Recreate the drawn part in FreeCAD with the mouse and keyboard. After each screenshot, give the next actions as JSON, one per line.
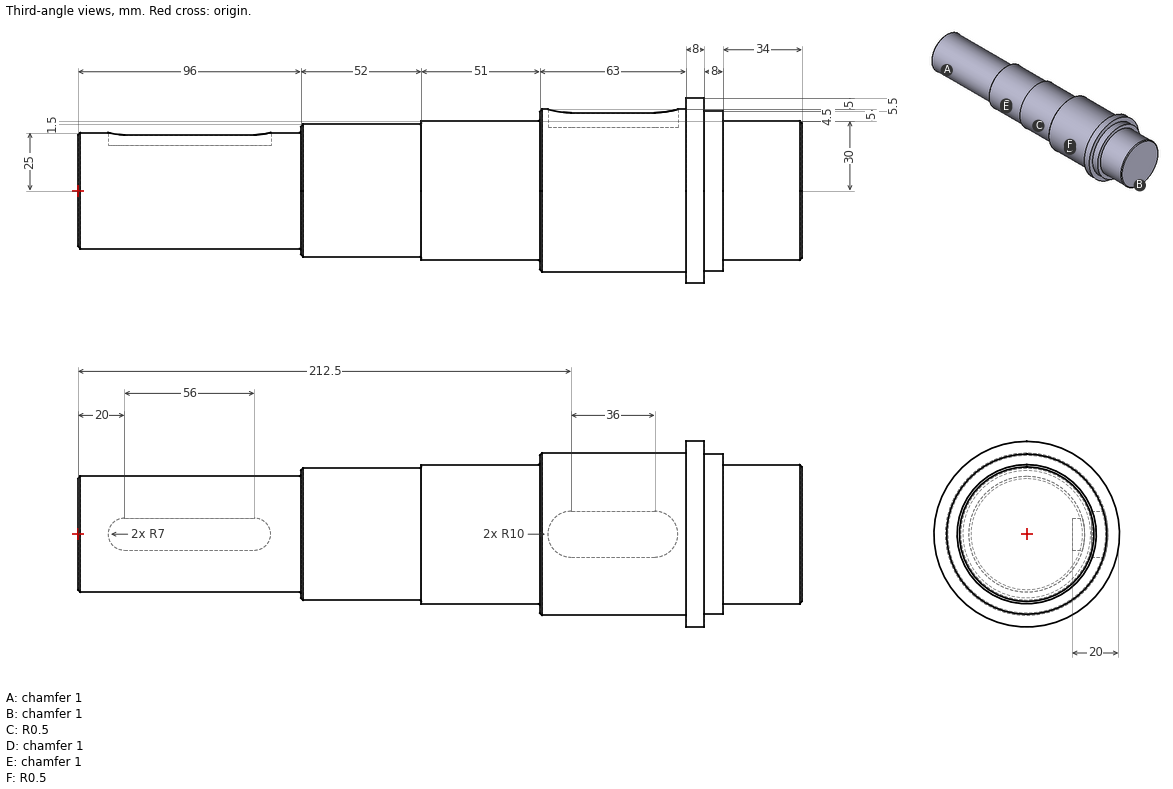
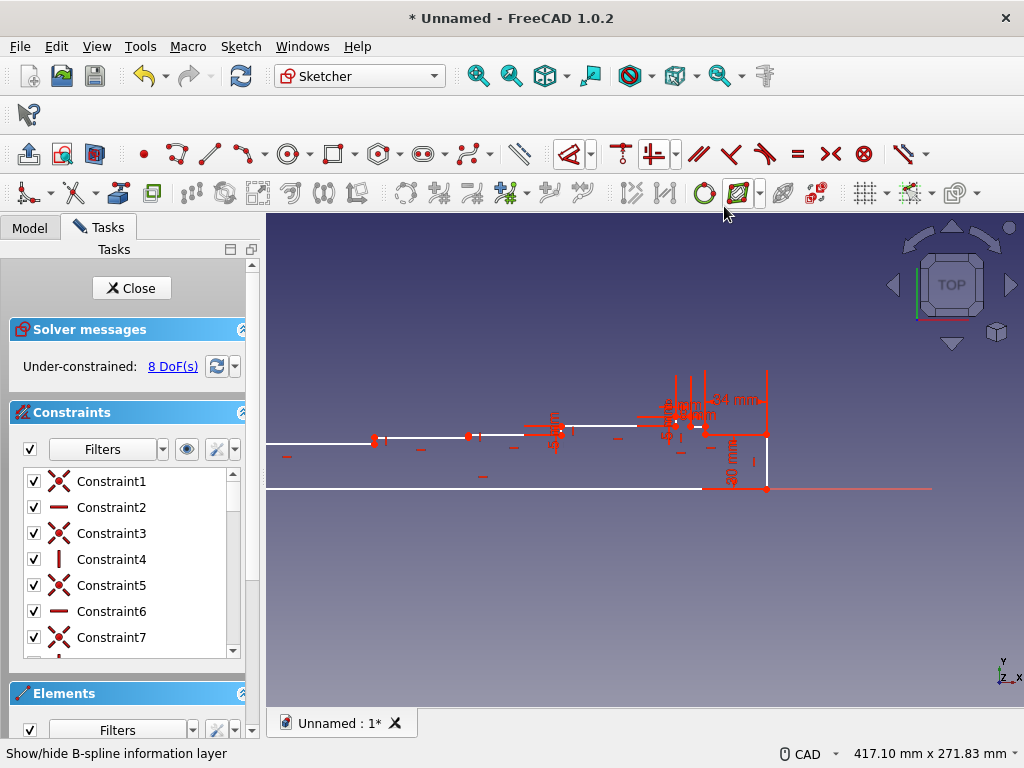
{"action": "left_click", "coordinate": [642, 426]}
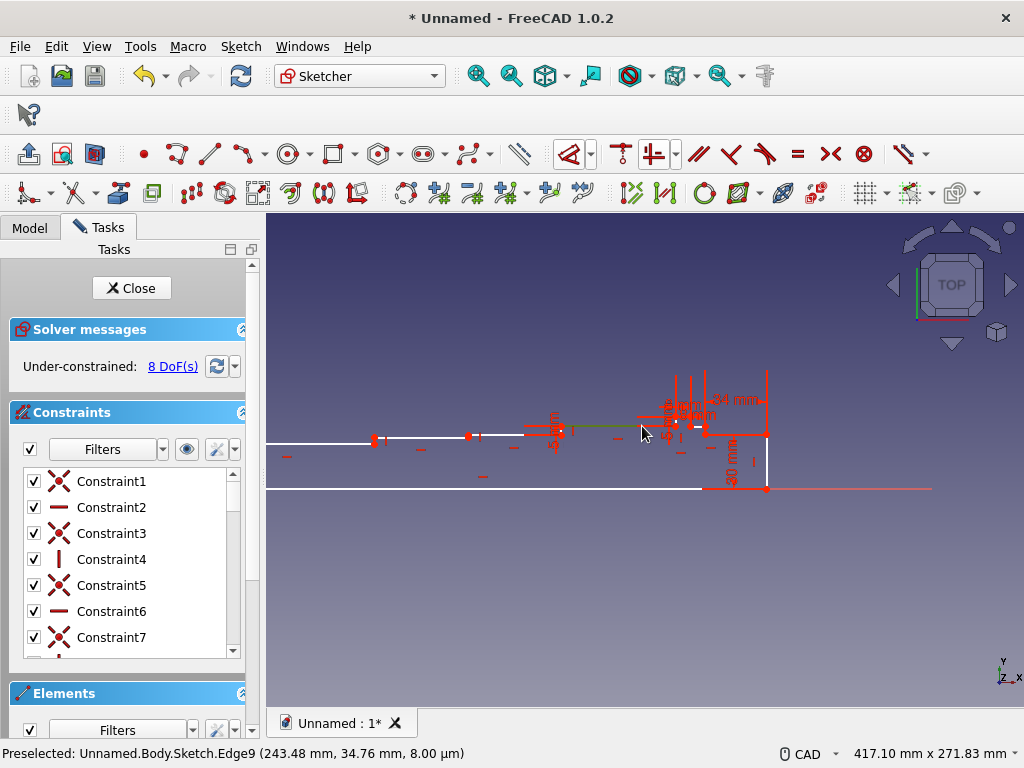
{"action": "key", "text": "l"}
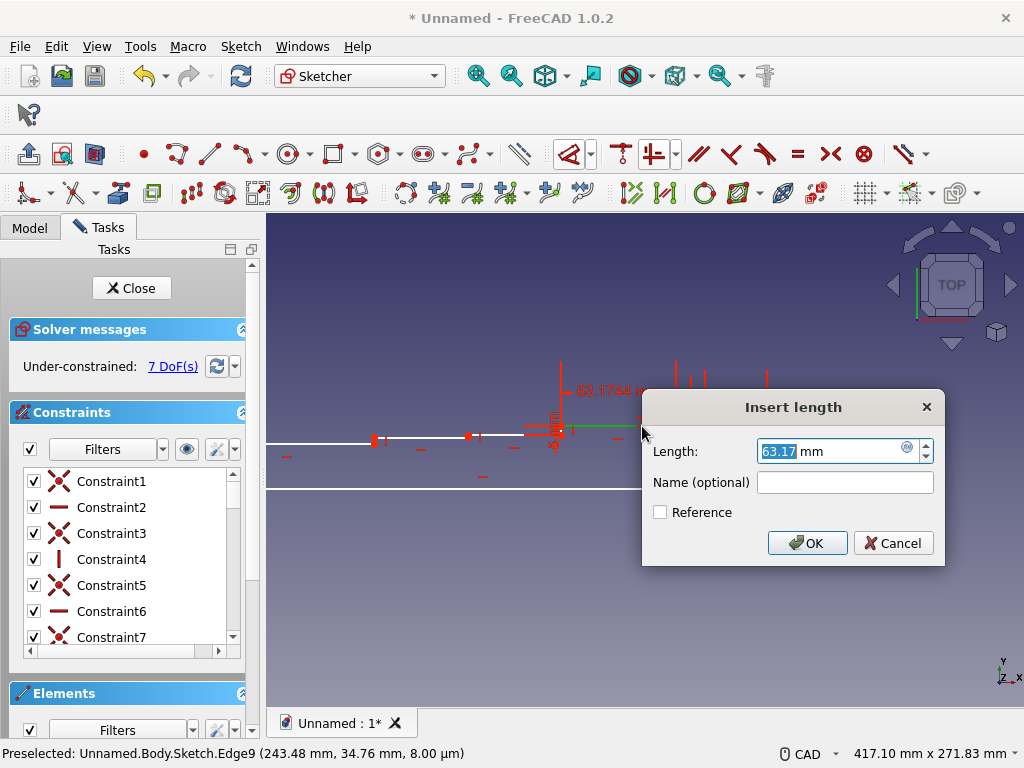
{"action": "type", "text": "63"}
{"action": "key", "text": "Return"}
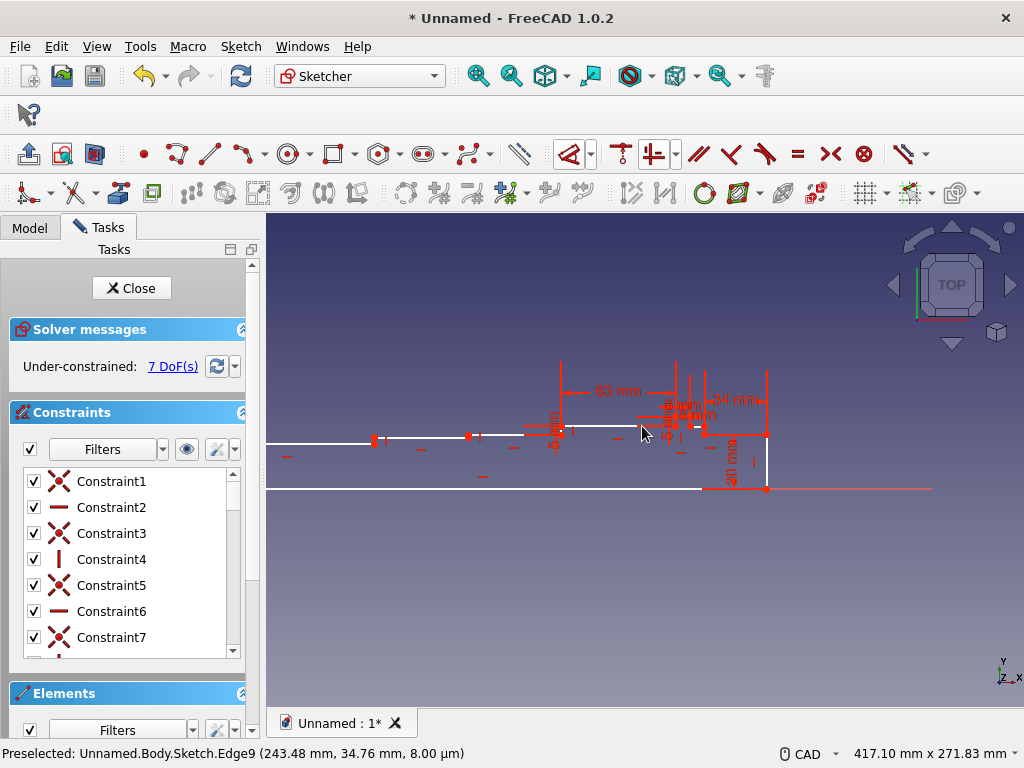
{"action": "left_click", "coordinate": [533, 435]}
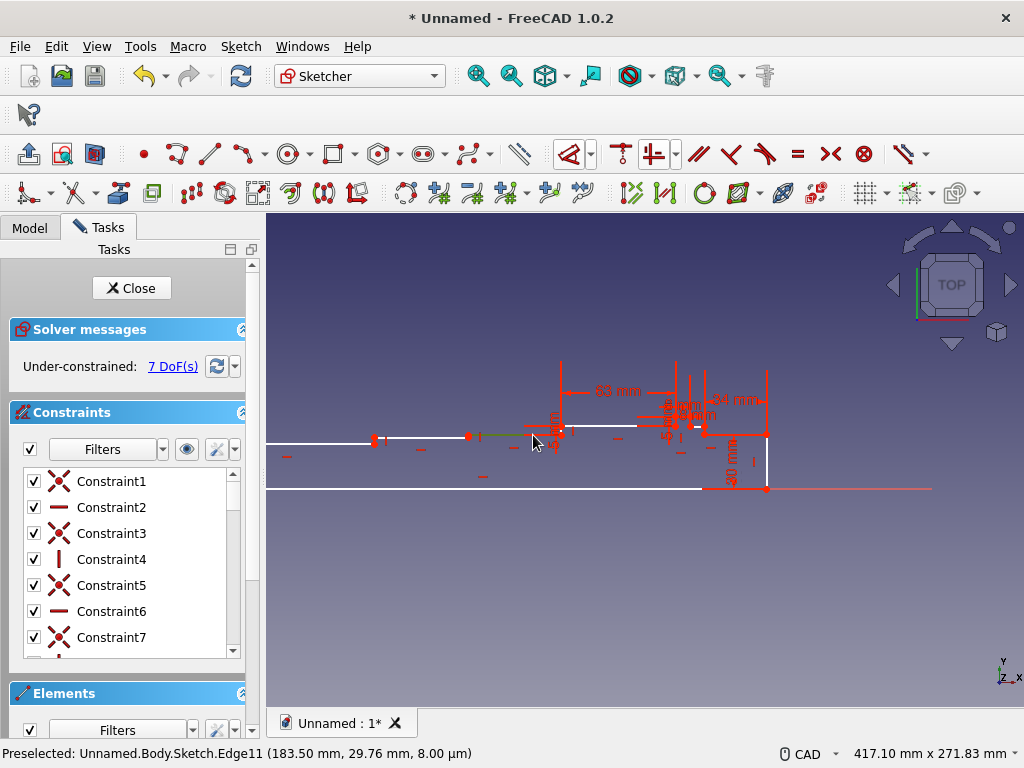
{"action": "key", "text": "l"}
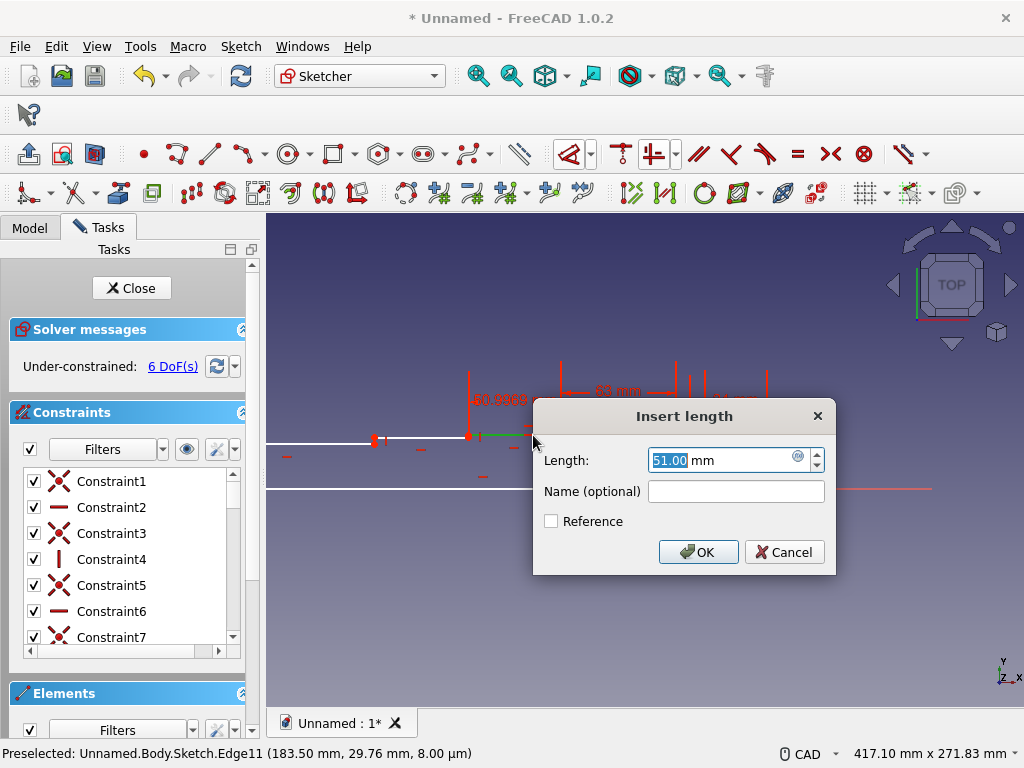
{"action": "type", "text": "51"}
{"action": "key", "text": "Return"}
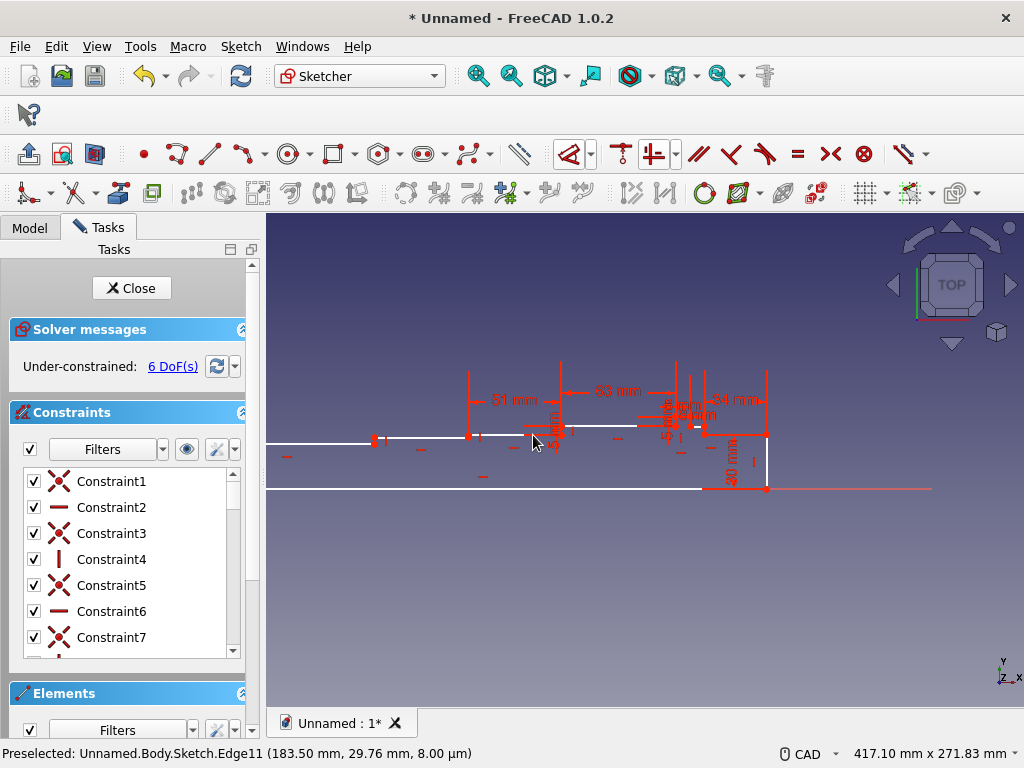
{"action": "left_click", "coordinate": [440, 438]}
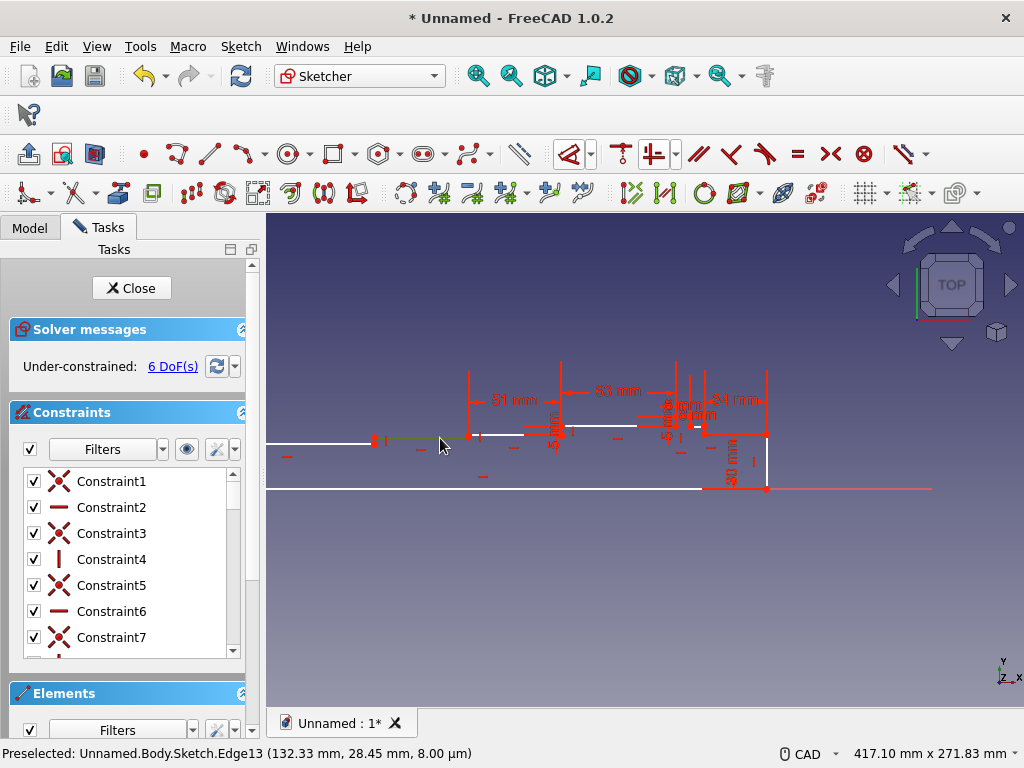
{"action": "key", "text": "l"}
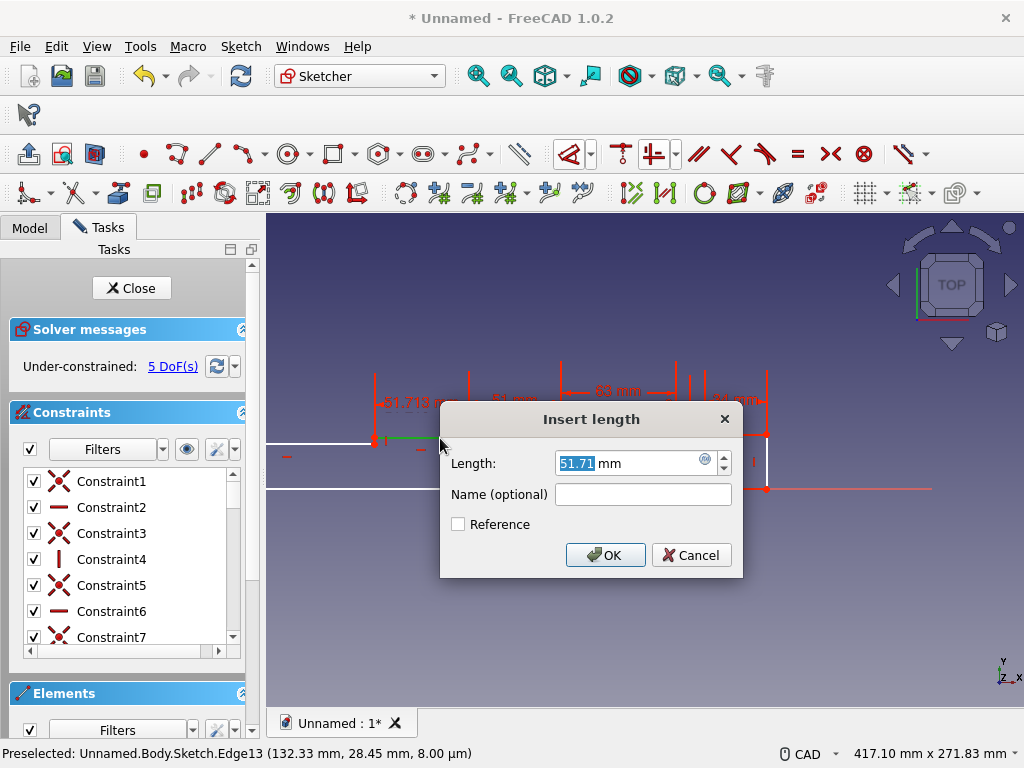
{"action": "type", "text": "52"}
{"action": "key", "text": "Return"}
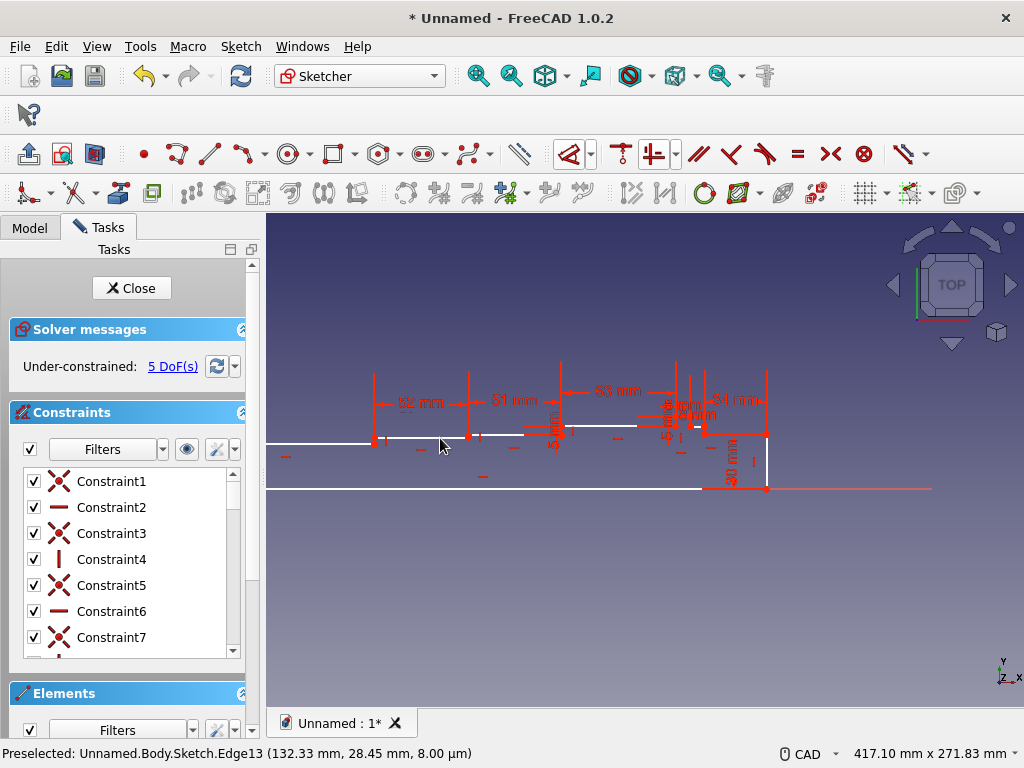
{"action": "left_click", "coordinate": [322, 444]}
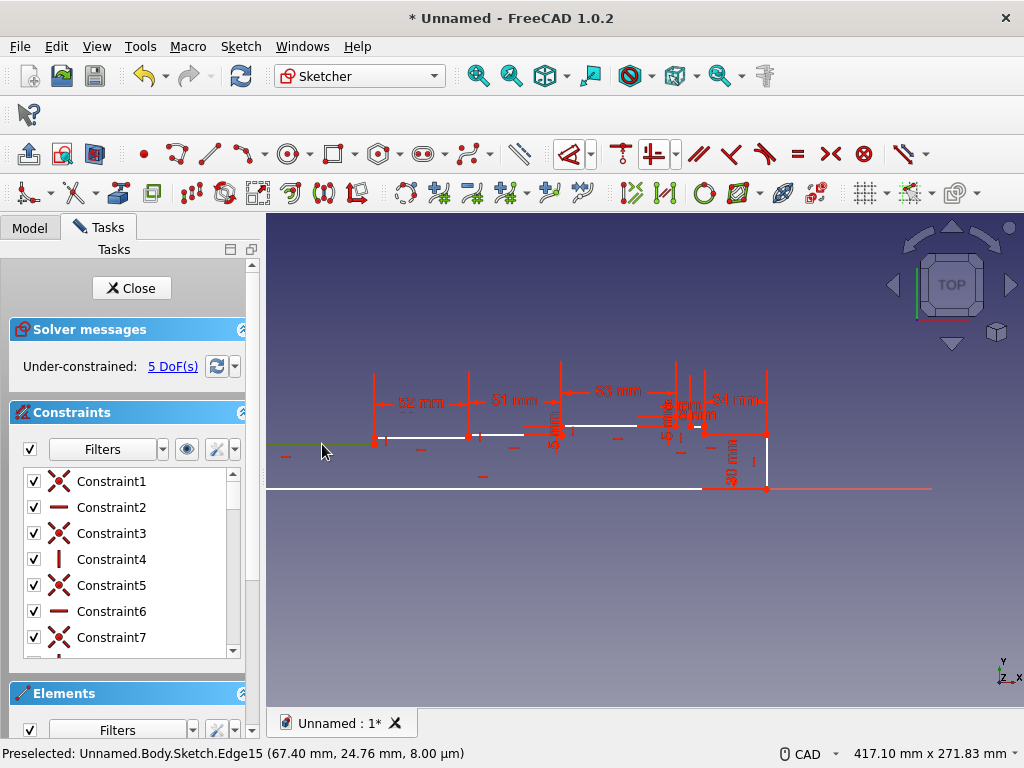
{"action": "key", "text": "l"}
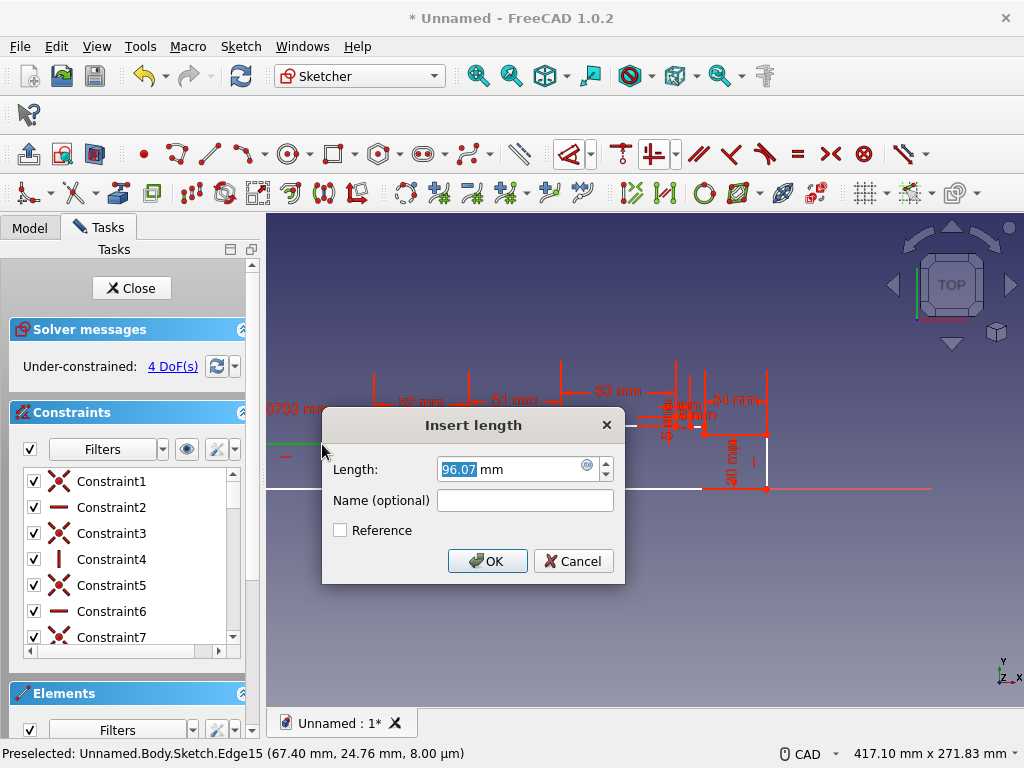
{"action": "type", "text": "96"}
{"action": "key", "text": "Return"}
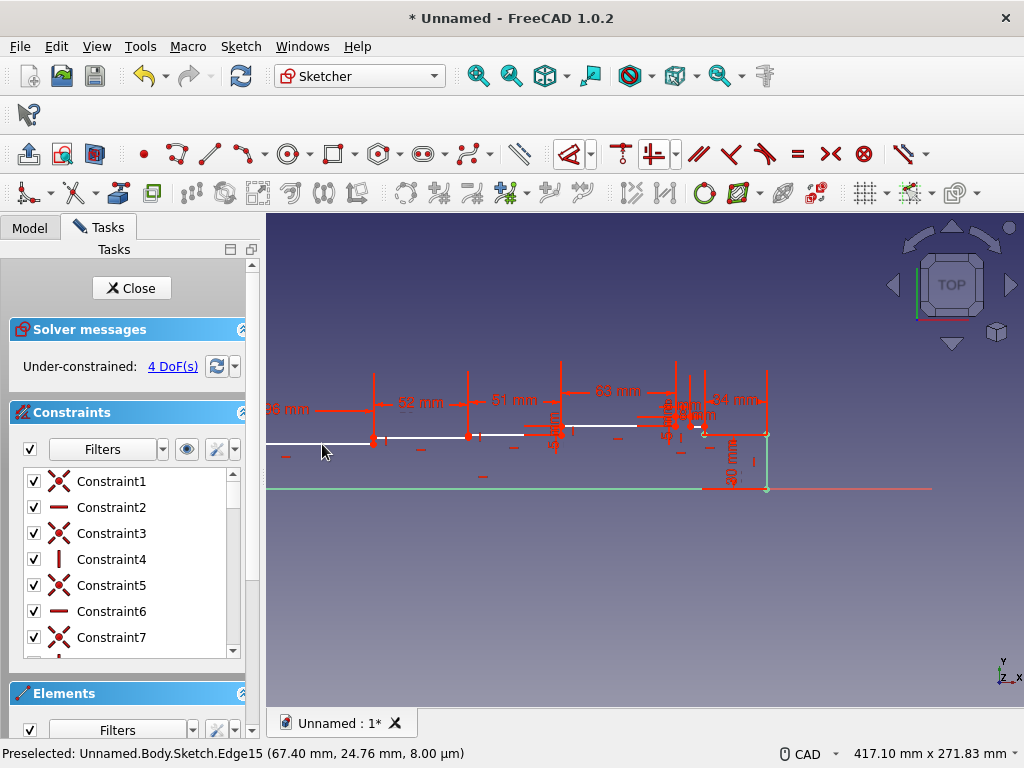
{"action": "scroll", "coordinate": [767, 474], "scroll_direction": "down", "scroll_amount": 2}